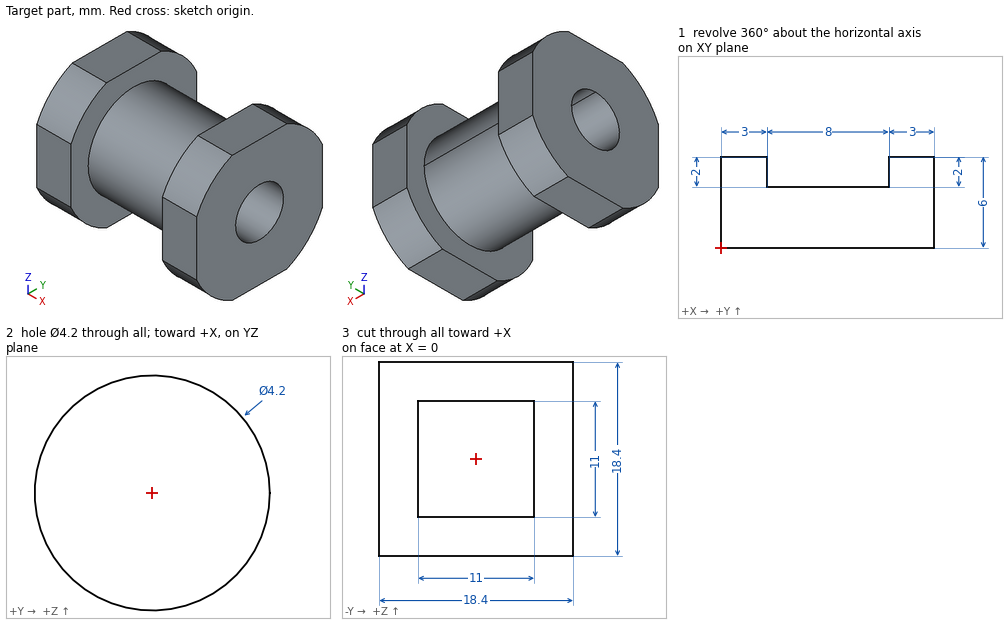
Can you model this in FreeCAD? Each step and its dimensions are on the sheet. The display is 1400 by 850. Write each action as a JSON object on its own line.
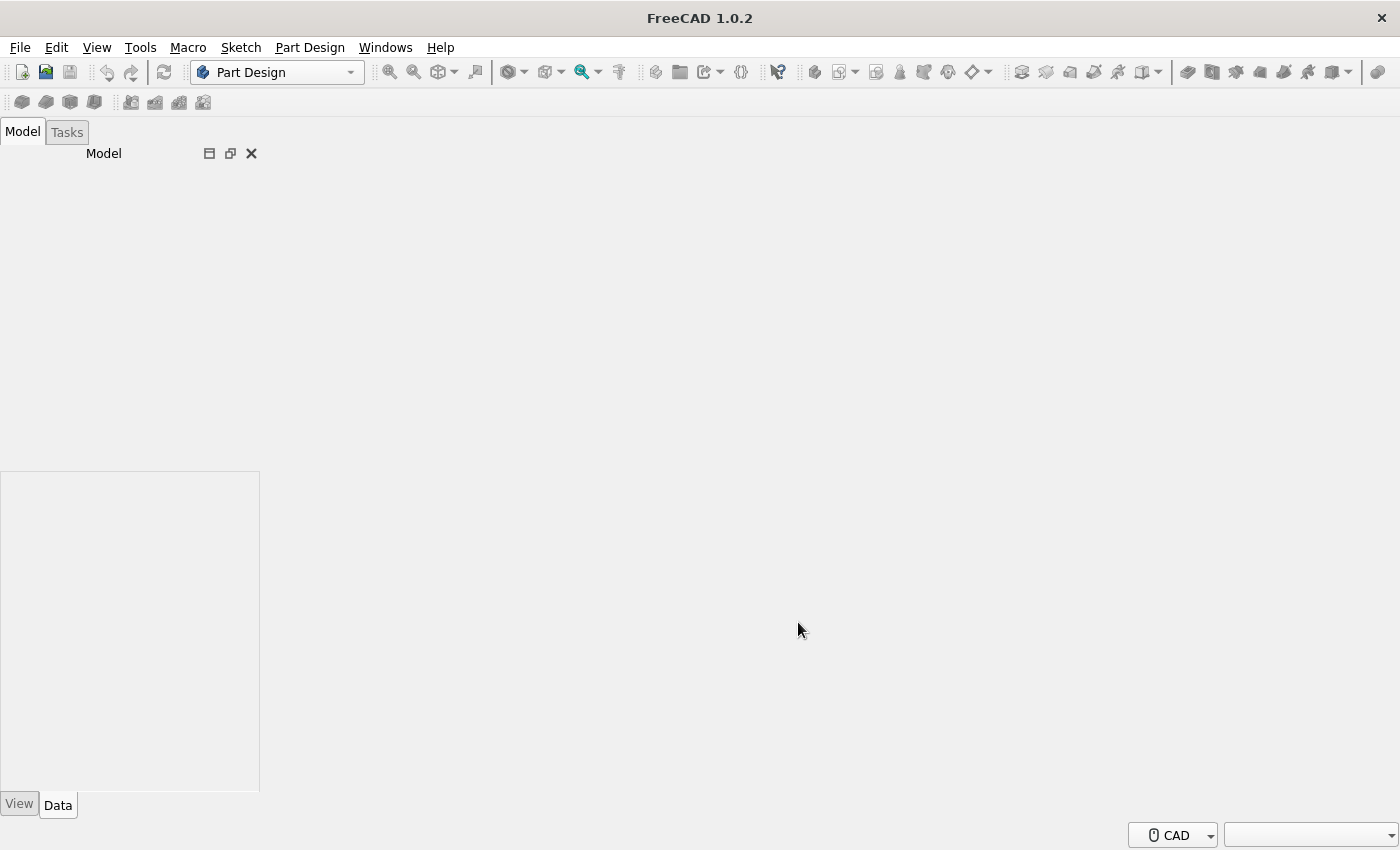
{"action": "left_click", "coordinate": [22, 72]}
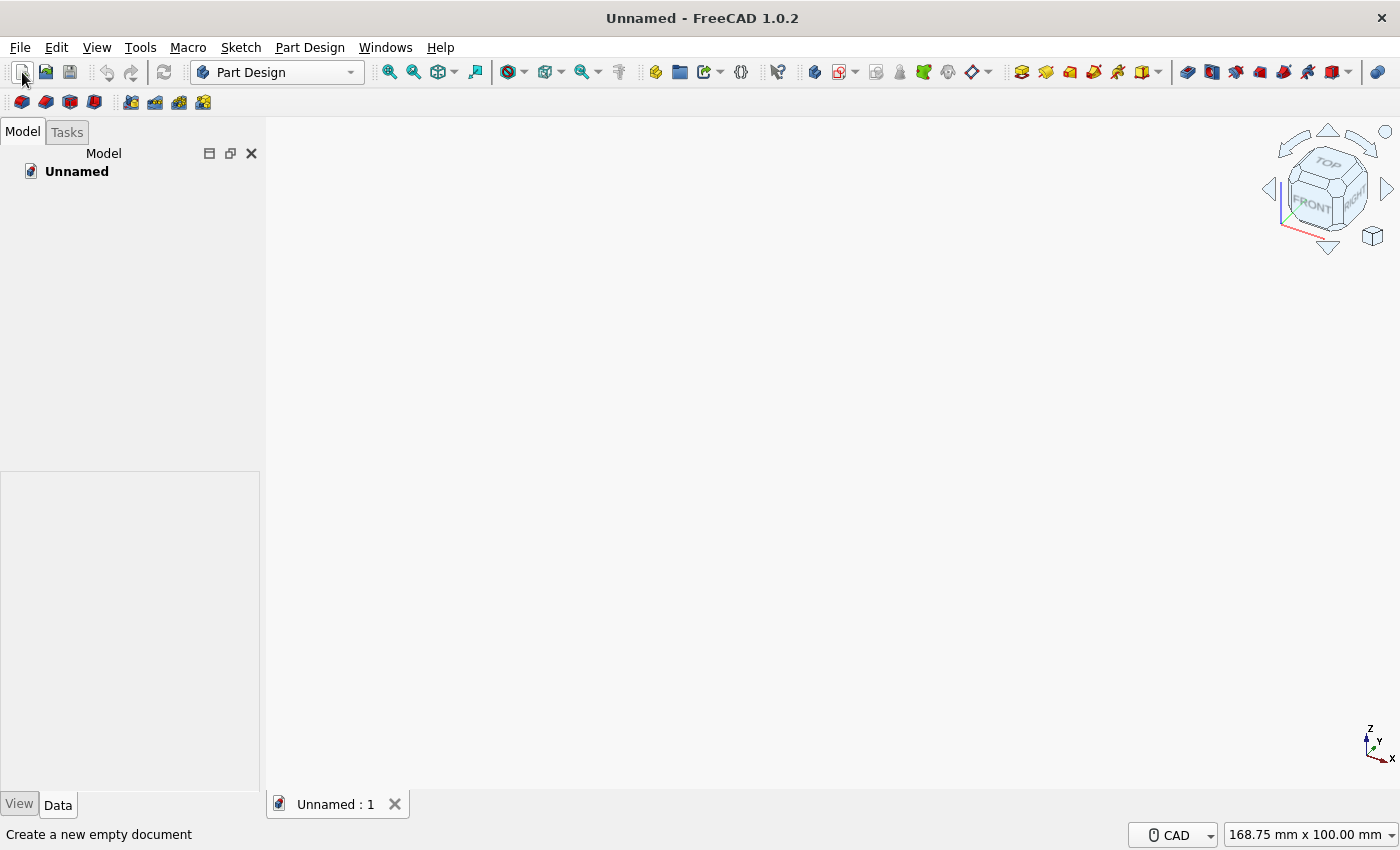
{"action": "left_click", "coordinate": [840, 72]}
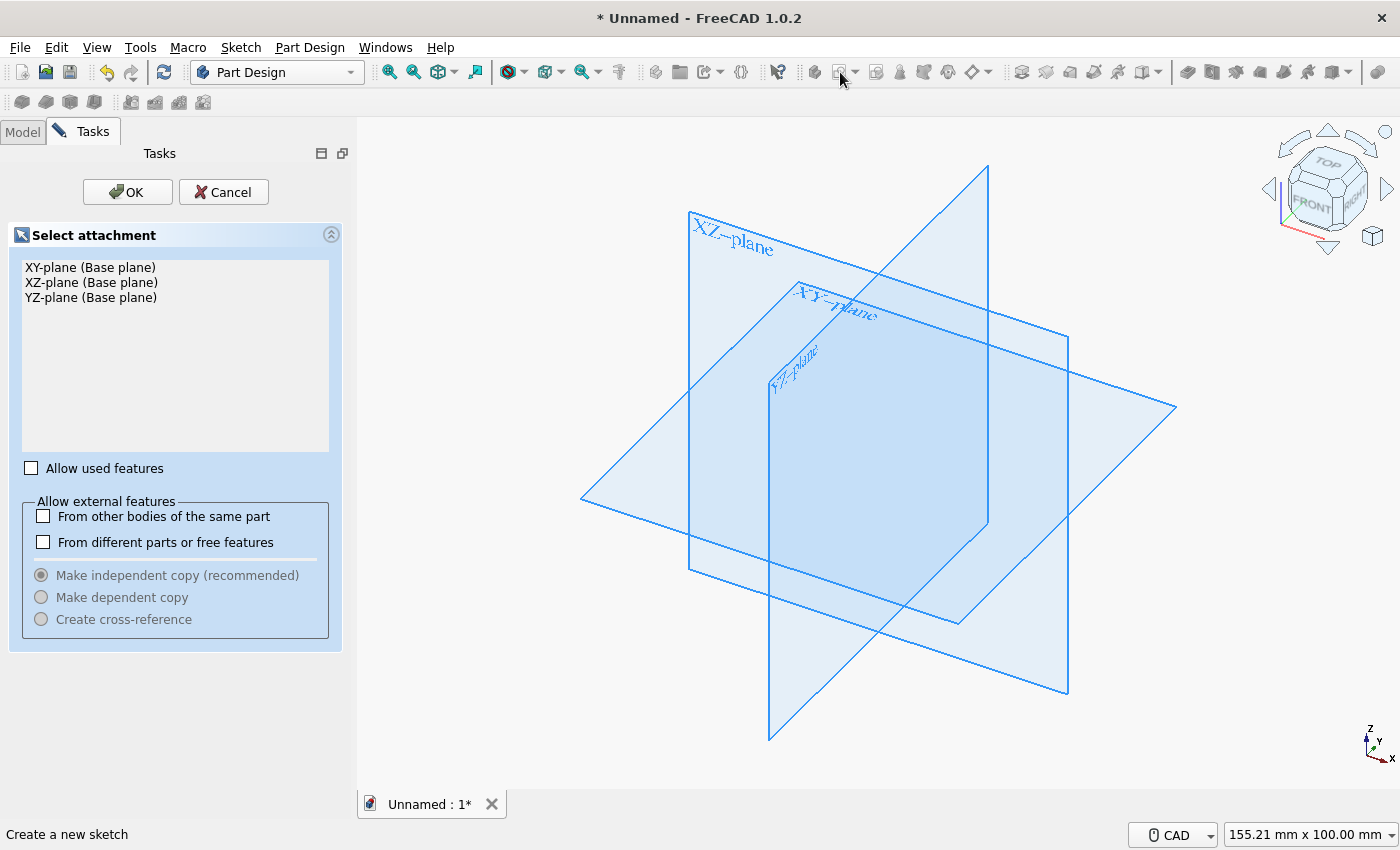
{"action": "left_click", "coordinate": [82, 268]}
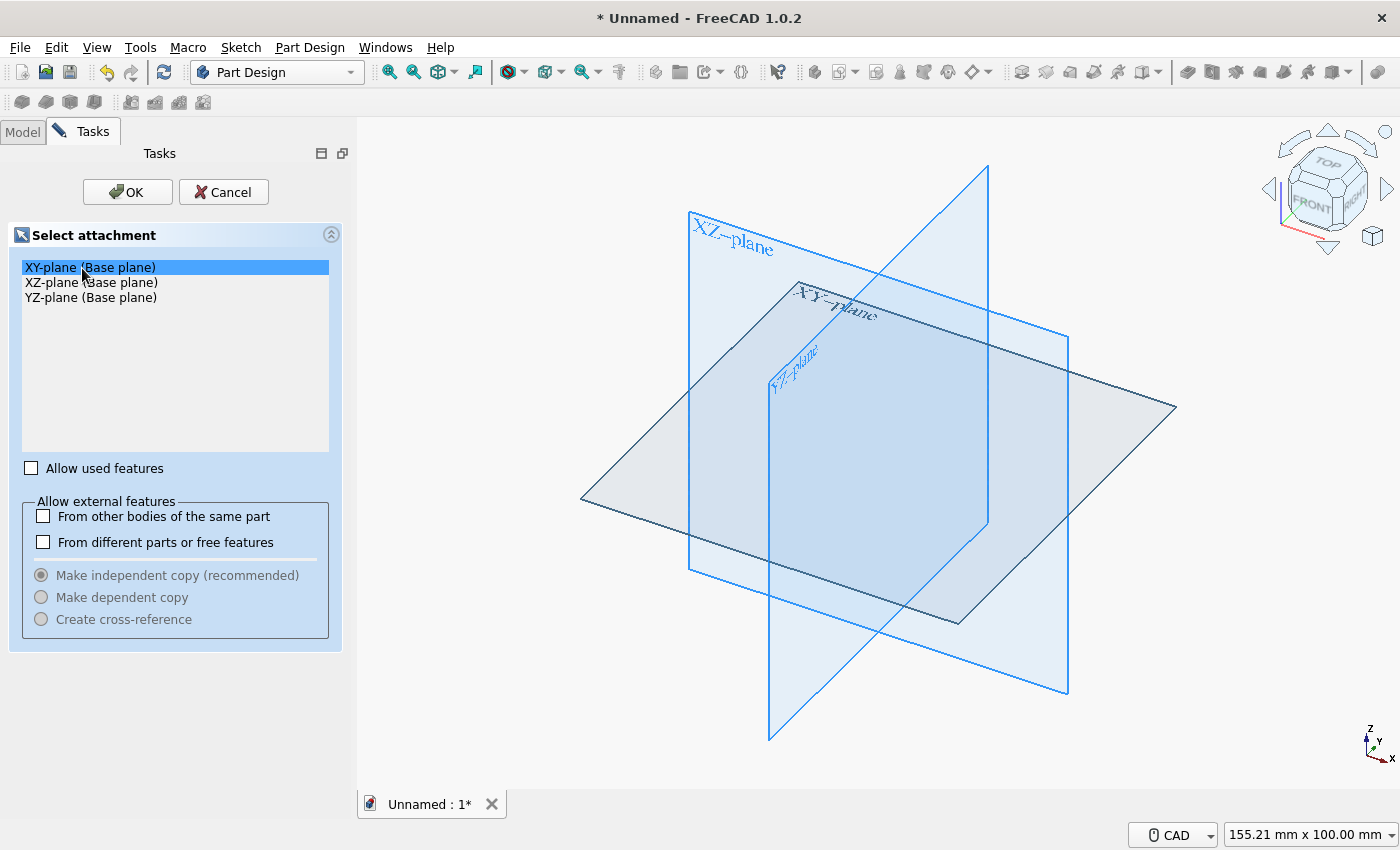
{"action": "left_click", "coordinate": [128, 192]}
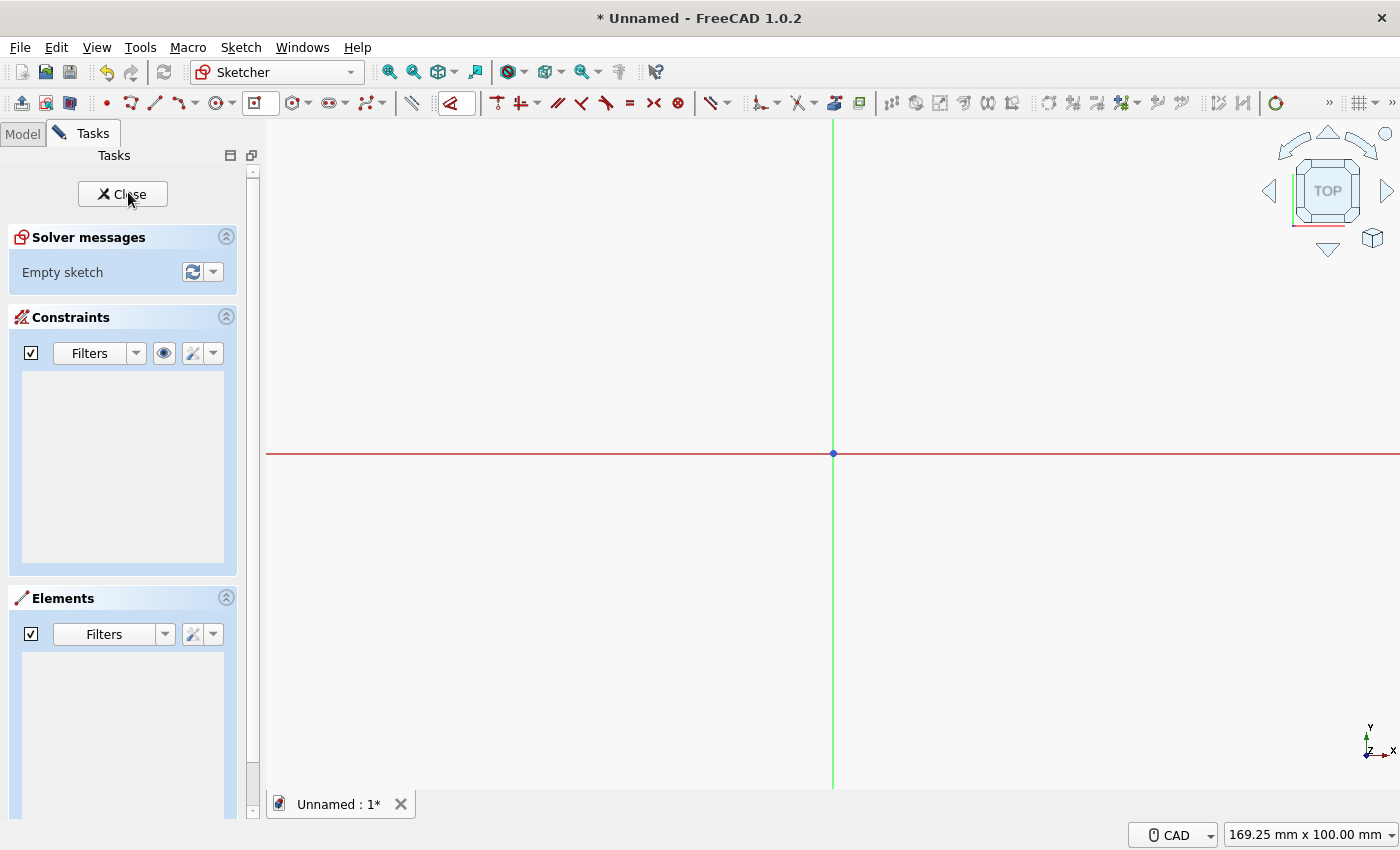
{"action": "scroll", "coordinate": [898, 431], "scroll_direction": "up", "scroll_amount": 10}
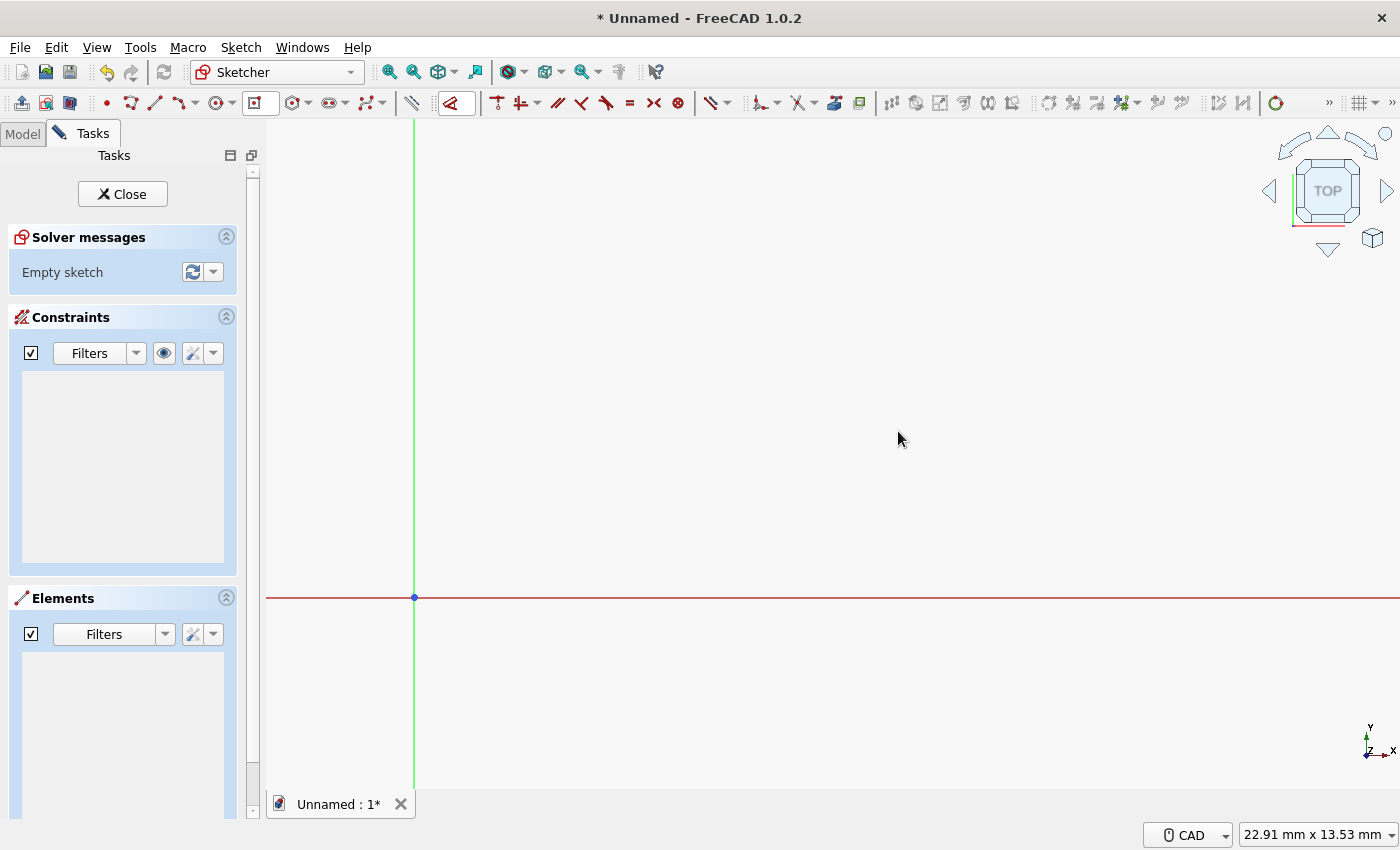
{"action": "left_click", "coordinate": [132, 104]}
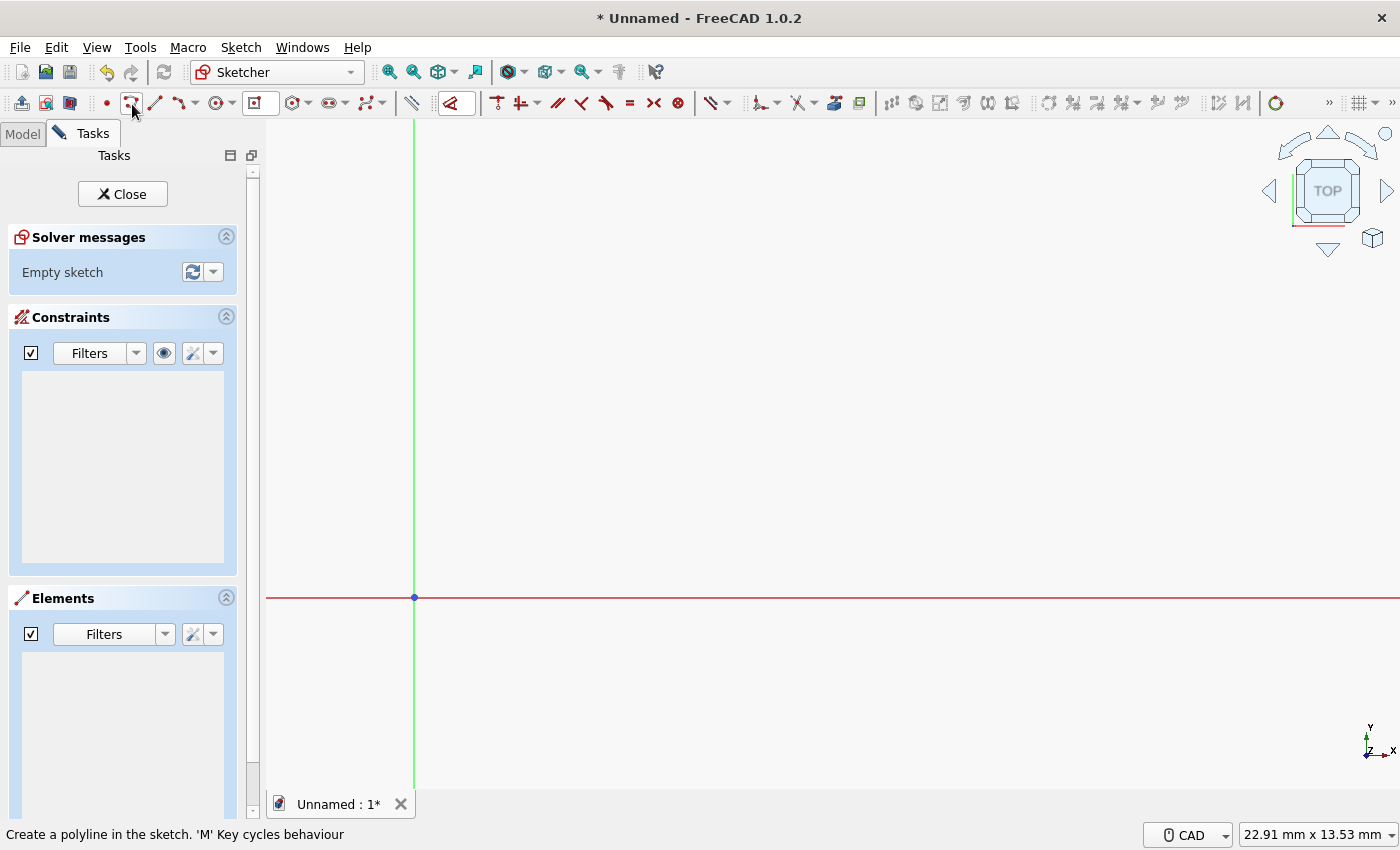
{"action": "left_click", "coordinate": [414, 598]}
{"action": "left_click", "coordinate": [1107, 589]}
{"action": "left_click", "coordinate": [1107, 301]}
{"action": "left_click", "coordinate": [959, 301]}
{"action": "left_click", "coordinate": [959, 400]}
{"action": "left_click", "coordinate": [563, 400]}
{"action": "left_click", "coordinate": [563, 301]}
{"action": "left_click", "coordinate": [423, 301]}
{"action": "left_click", "coordinate": [414, 598]}
{"action": "key", "text": "Escape"}
{"action": "key", "text": "Escape"}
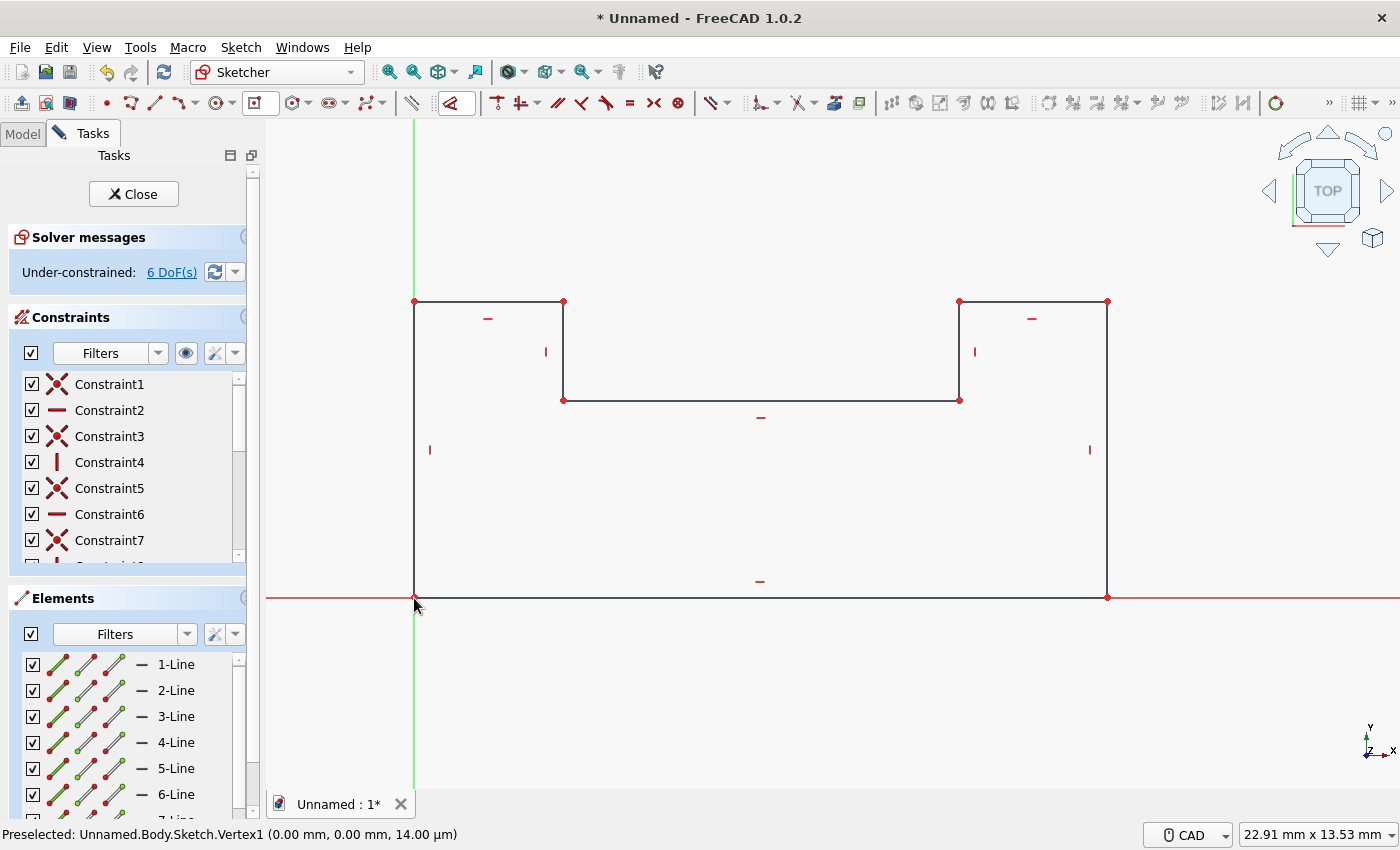
{"action": "left_click", "coordinate": [1107, 509]}